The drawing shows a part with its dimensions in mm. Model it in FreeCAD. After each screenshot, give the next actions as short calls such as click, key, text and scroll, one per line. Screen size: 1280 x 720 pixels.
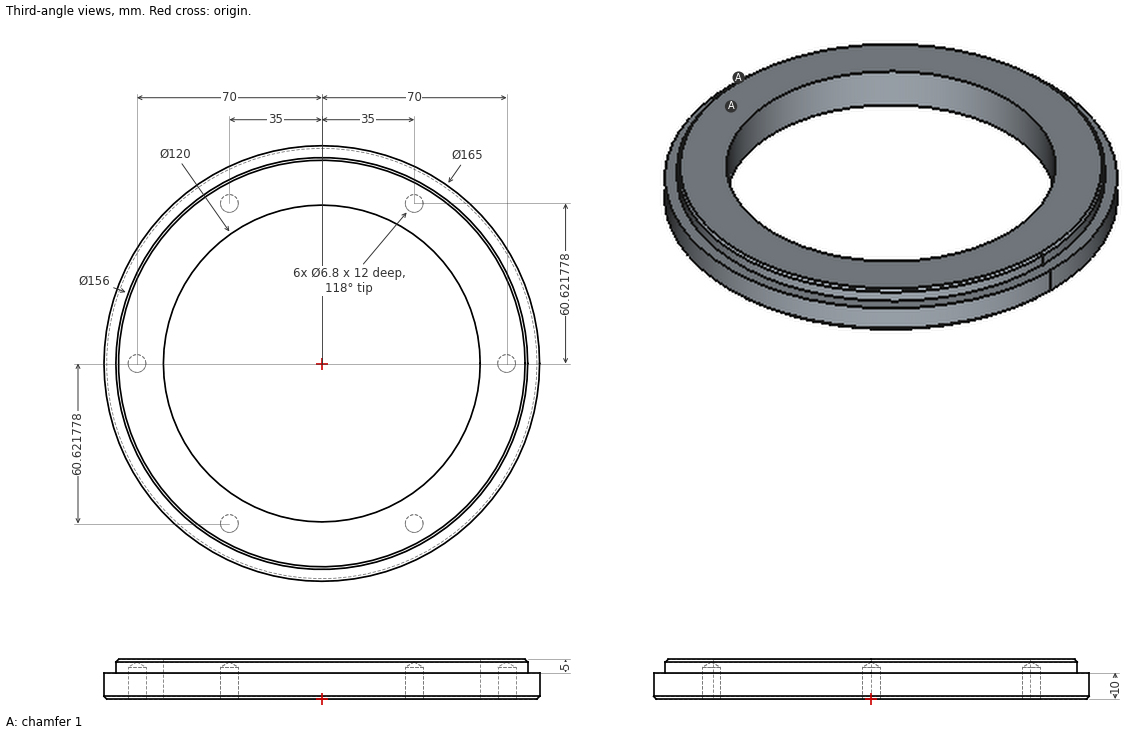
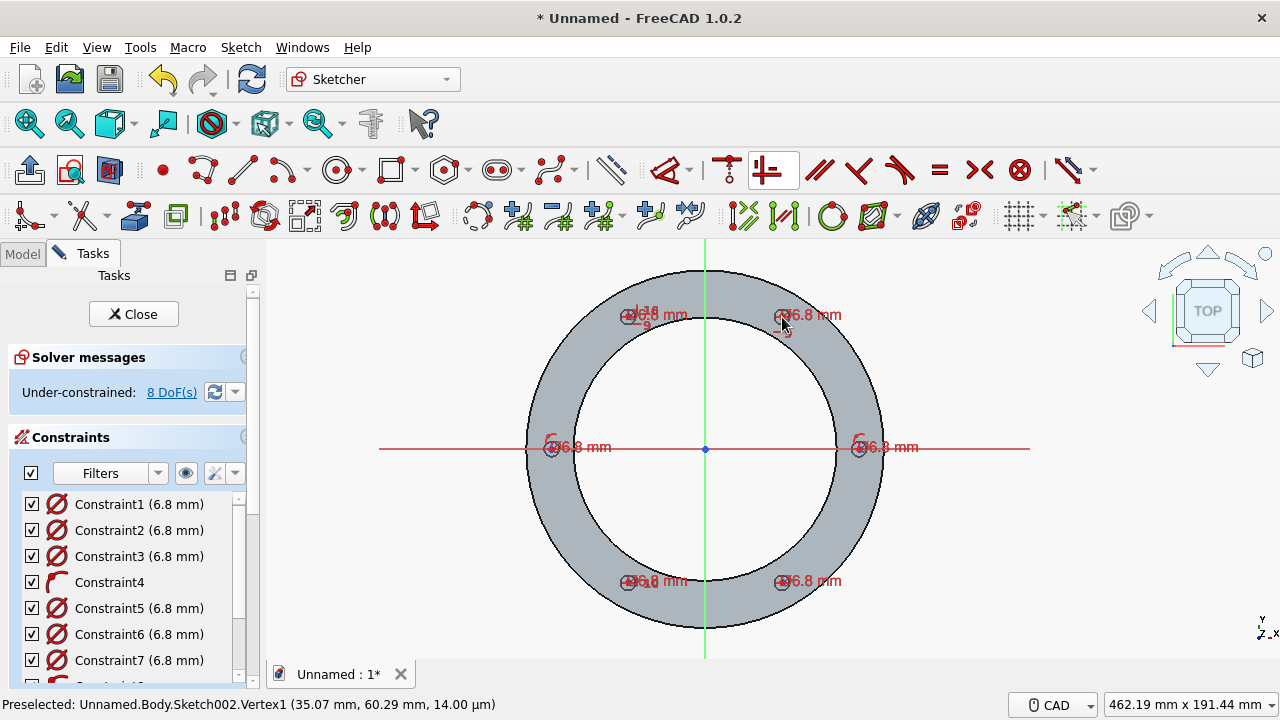
click(782, 583)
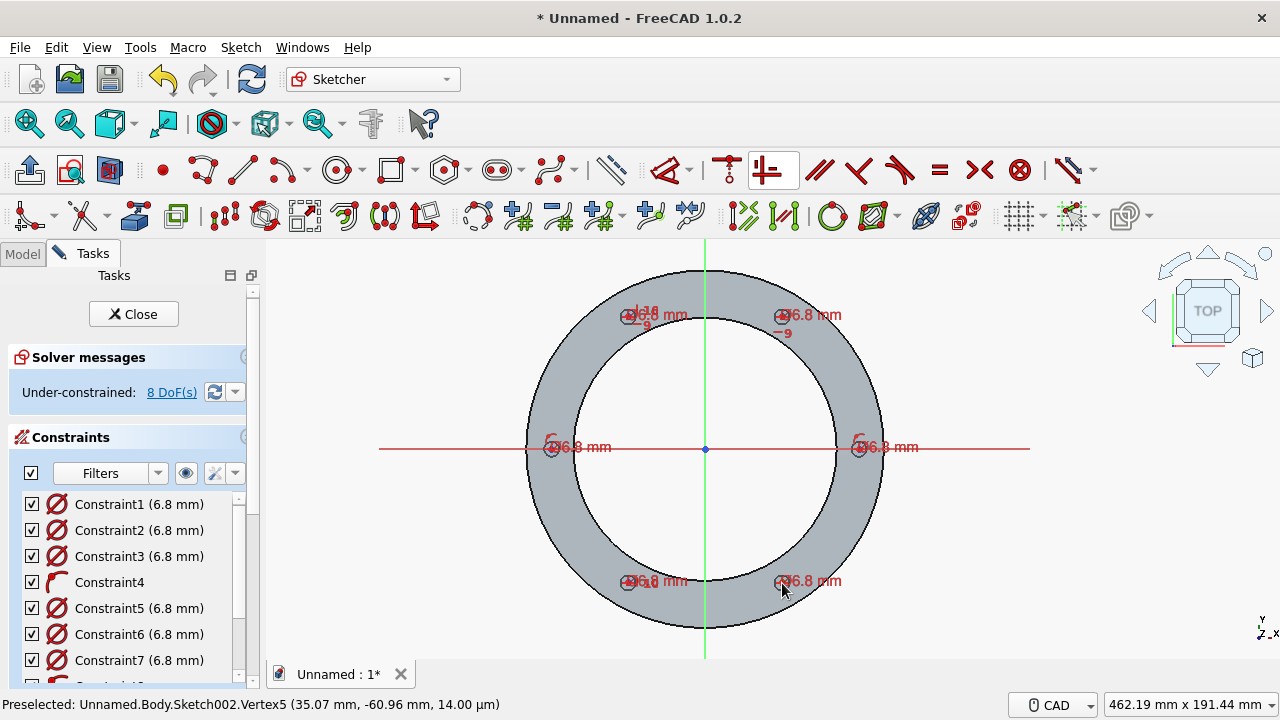
key(v)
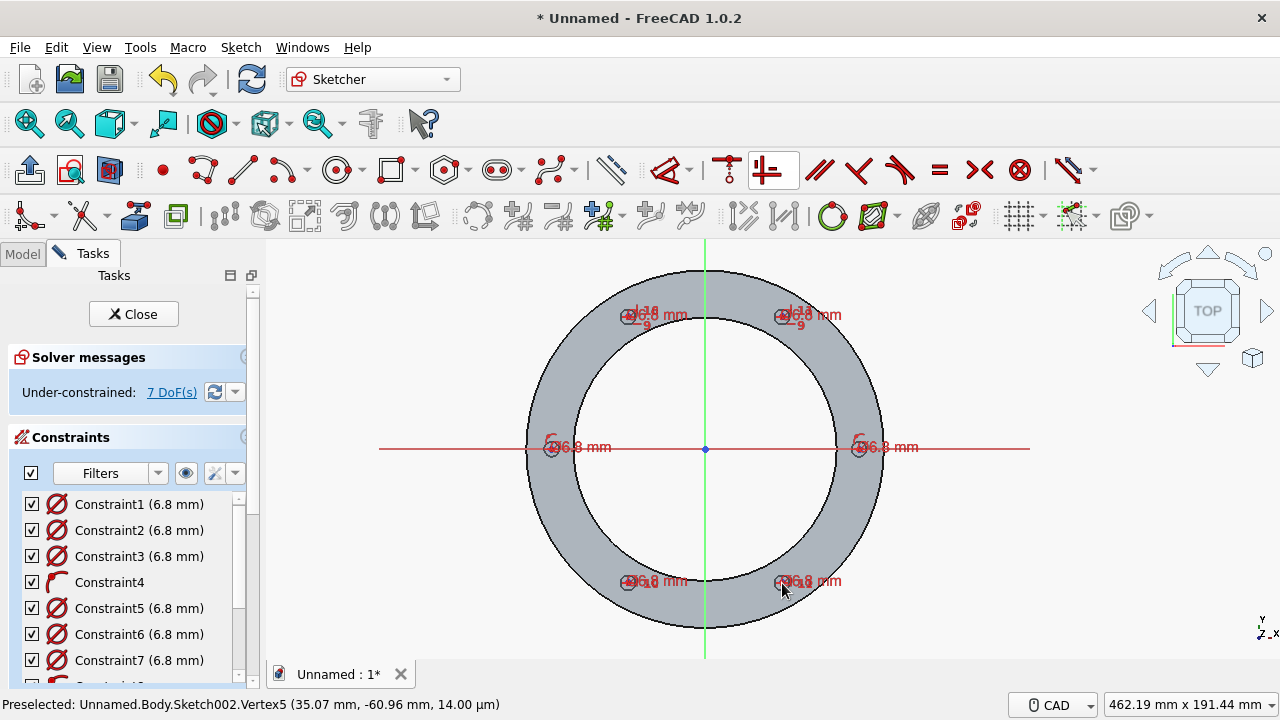
click(628, 583)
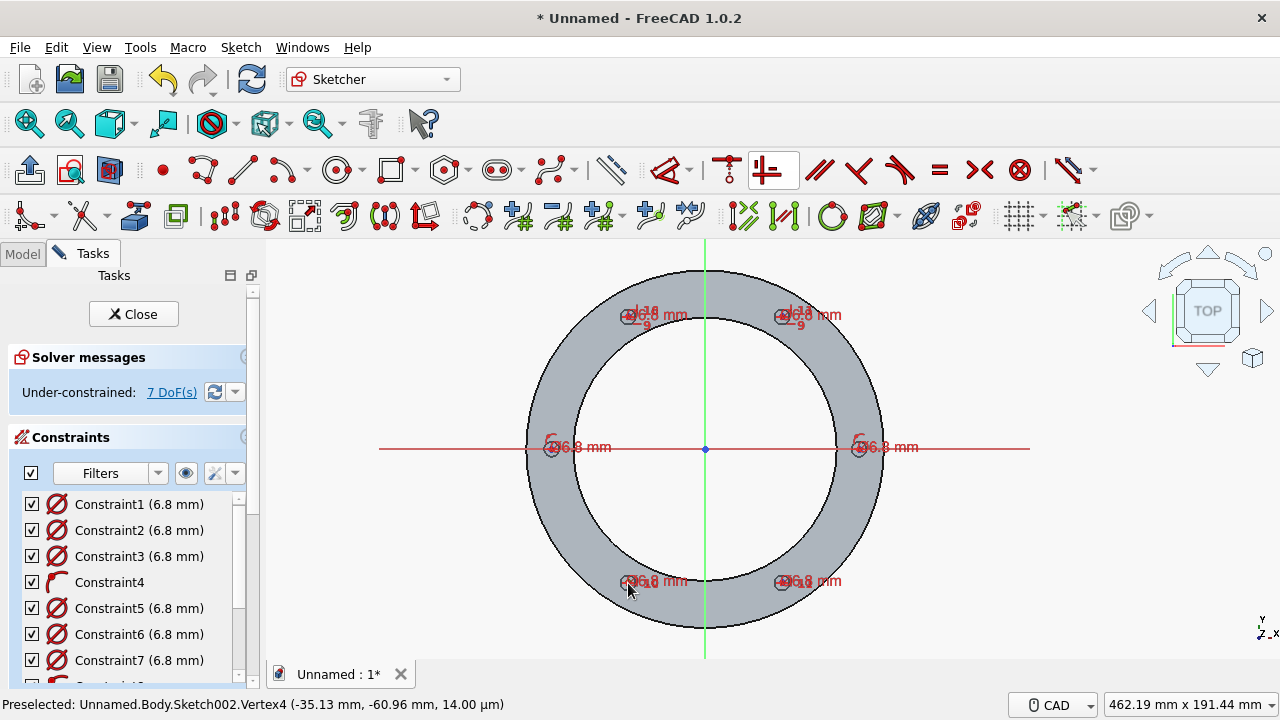
click(782, 583)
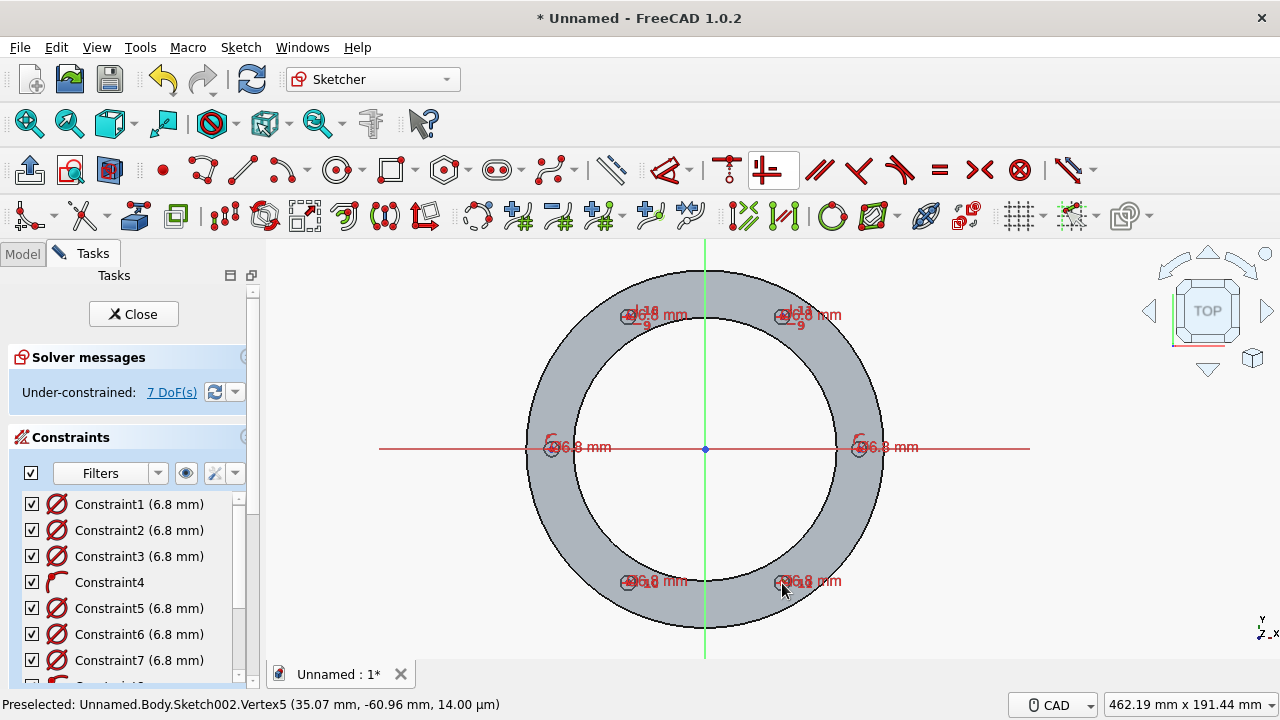
key(h)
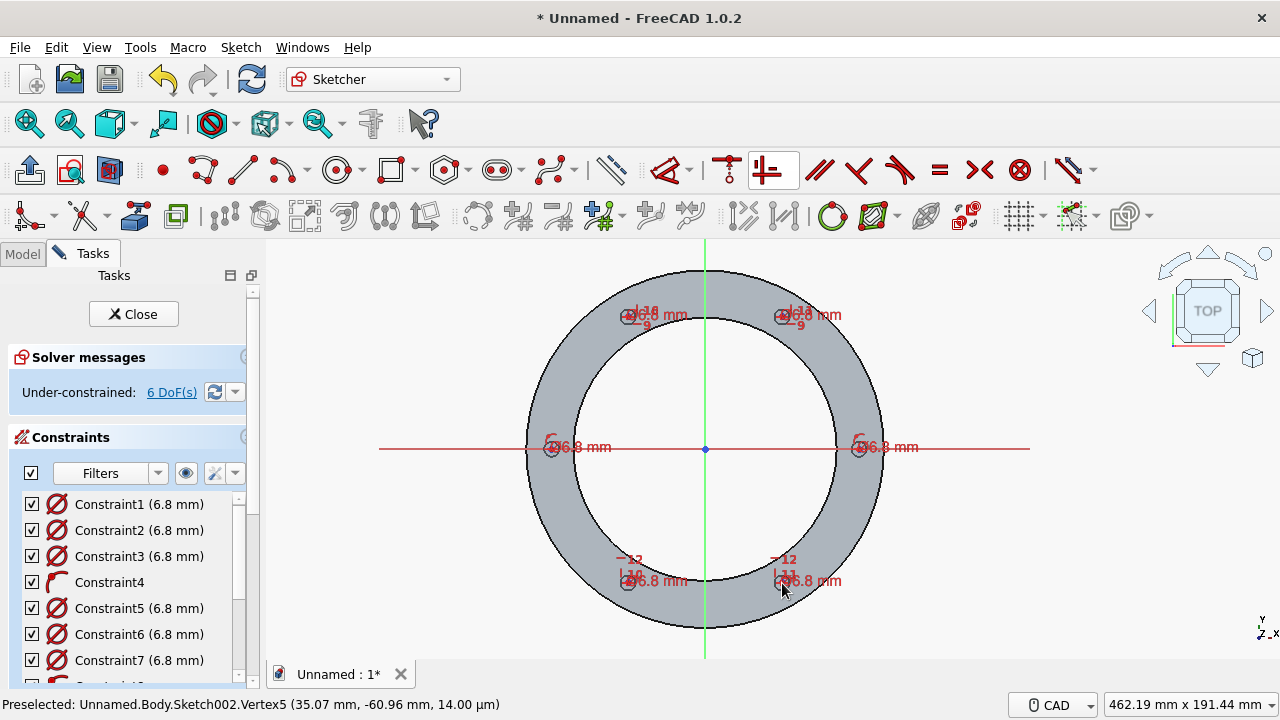
click(782, 317)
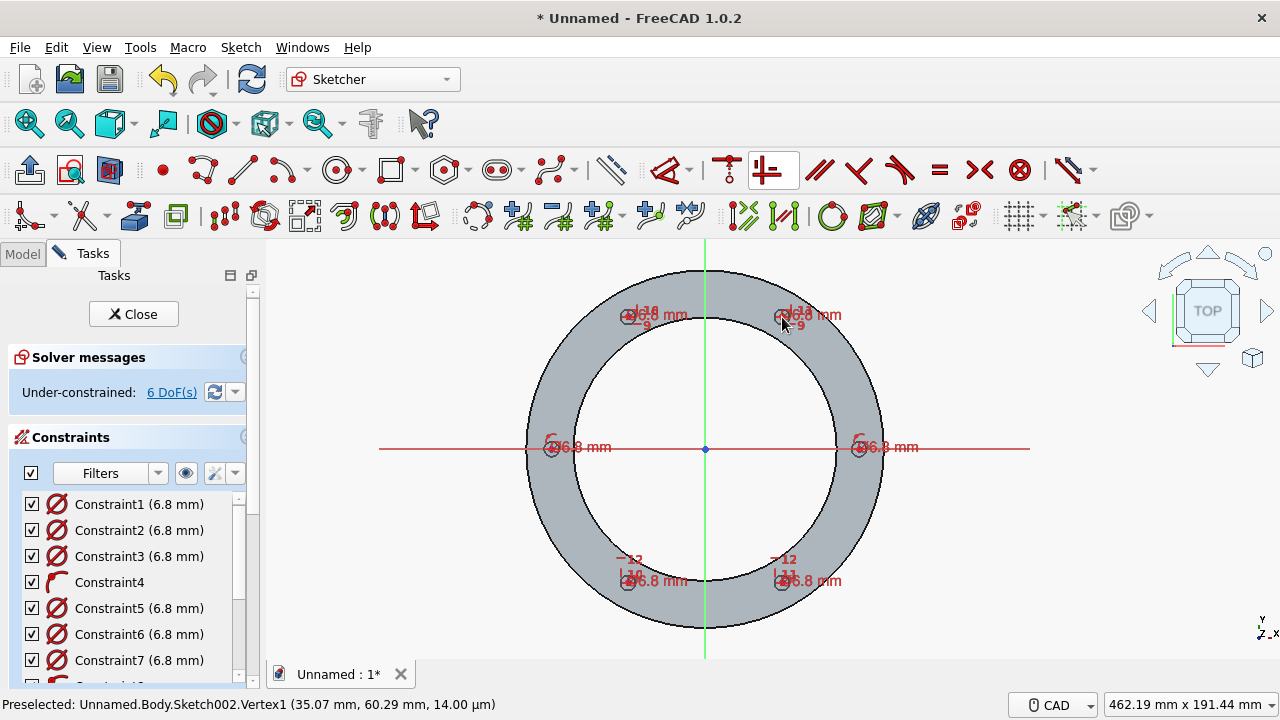
click(692, 170)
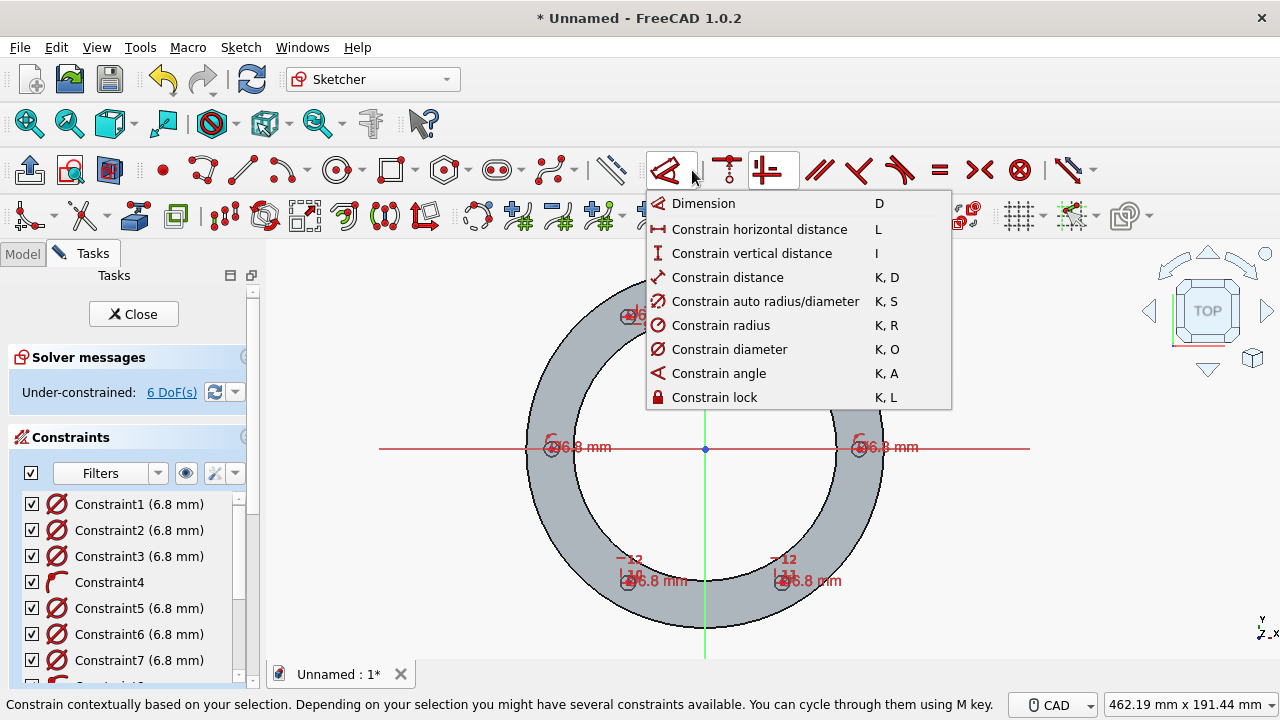
click(799, 229)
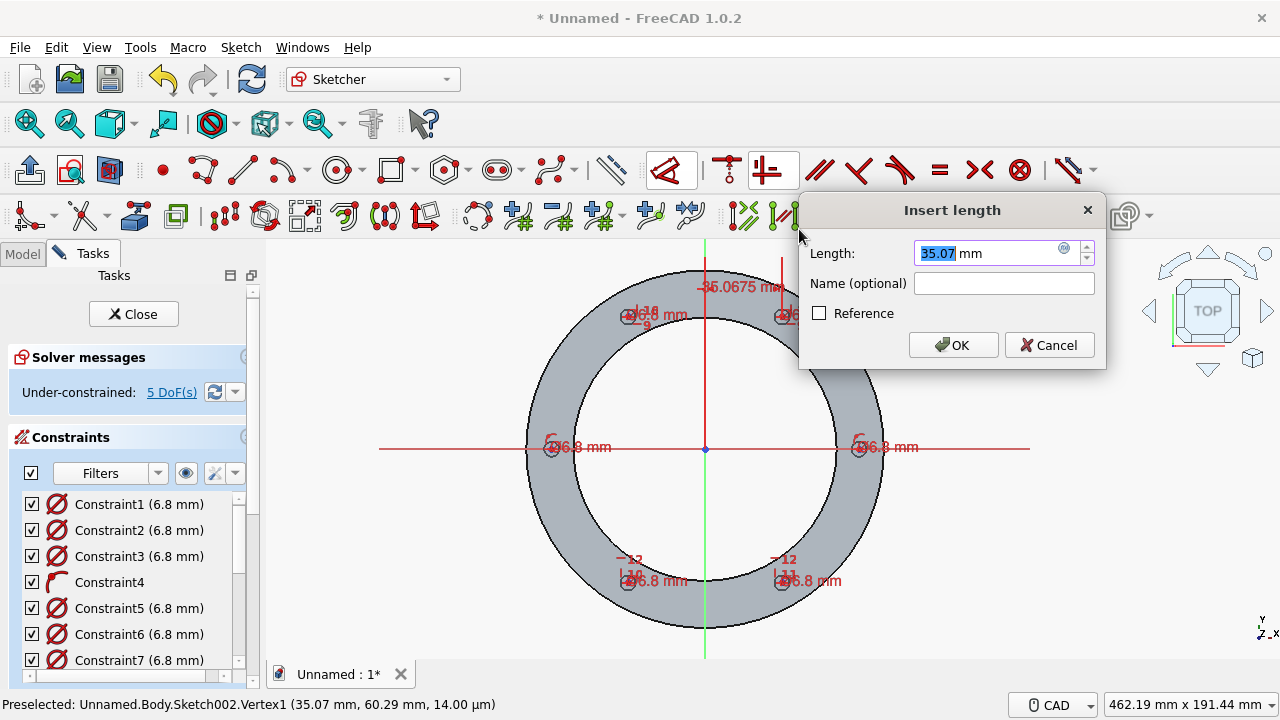
text(35)
key(Return)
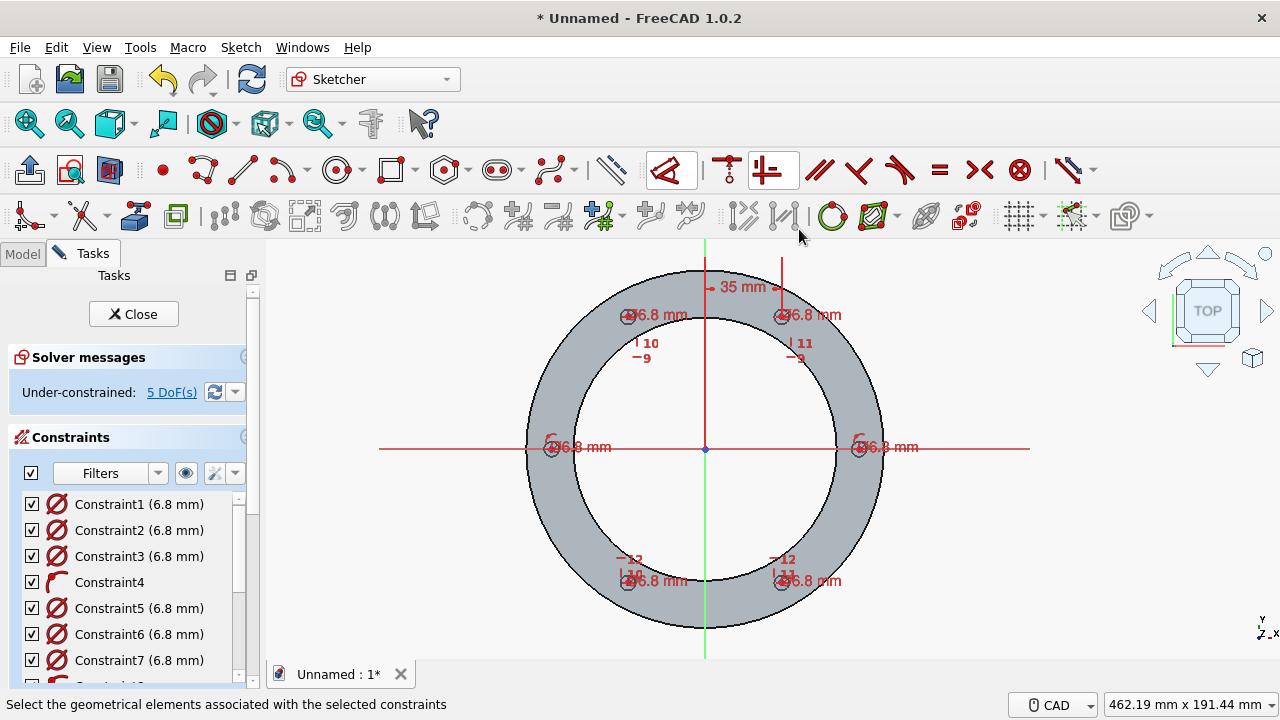
click(628, 317)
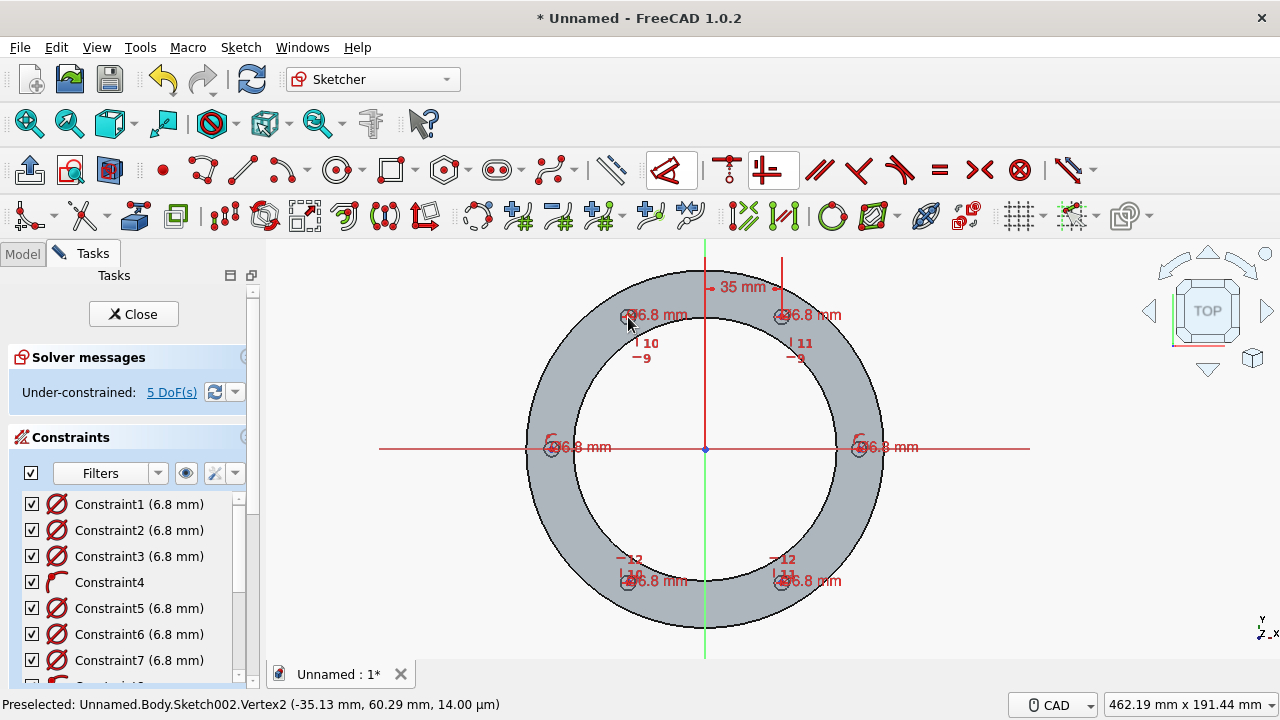
click(692, 170)